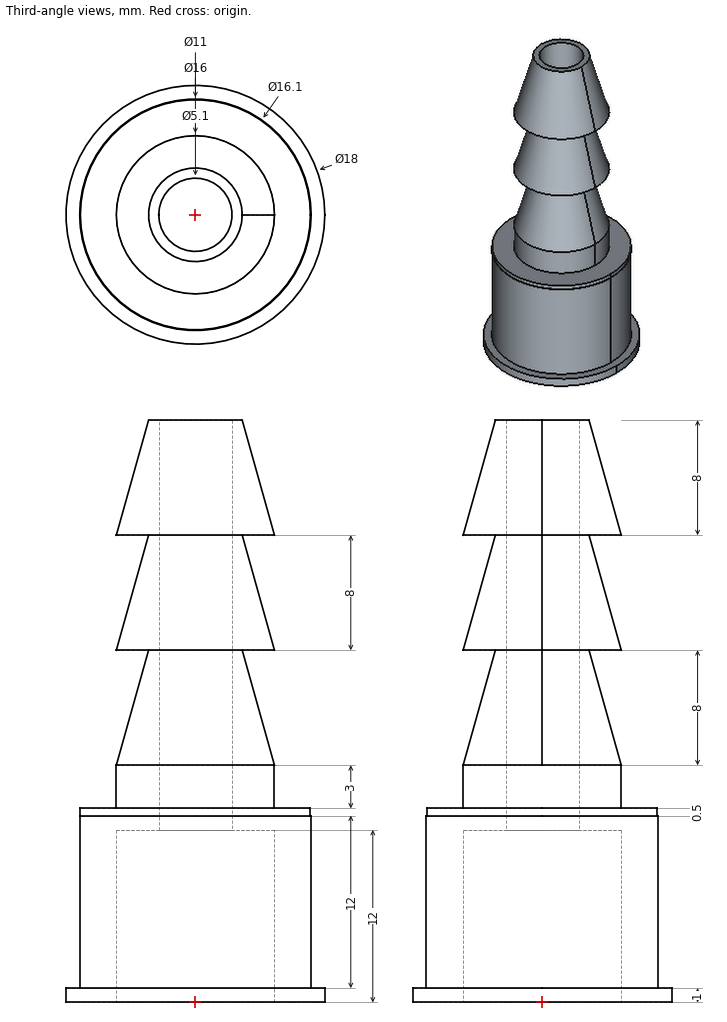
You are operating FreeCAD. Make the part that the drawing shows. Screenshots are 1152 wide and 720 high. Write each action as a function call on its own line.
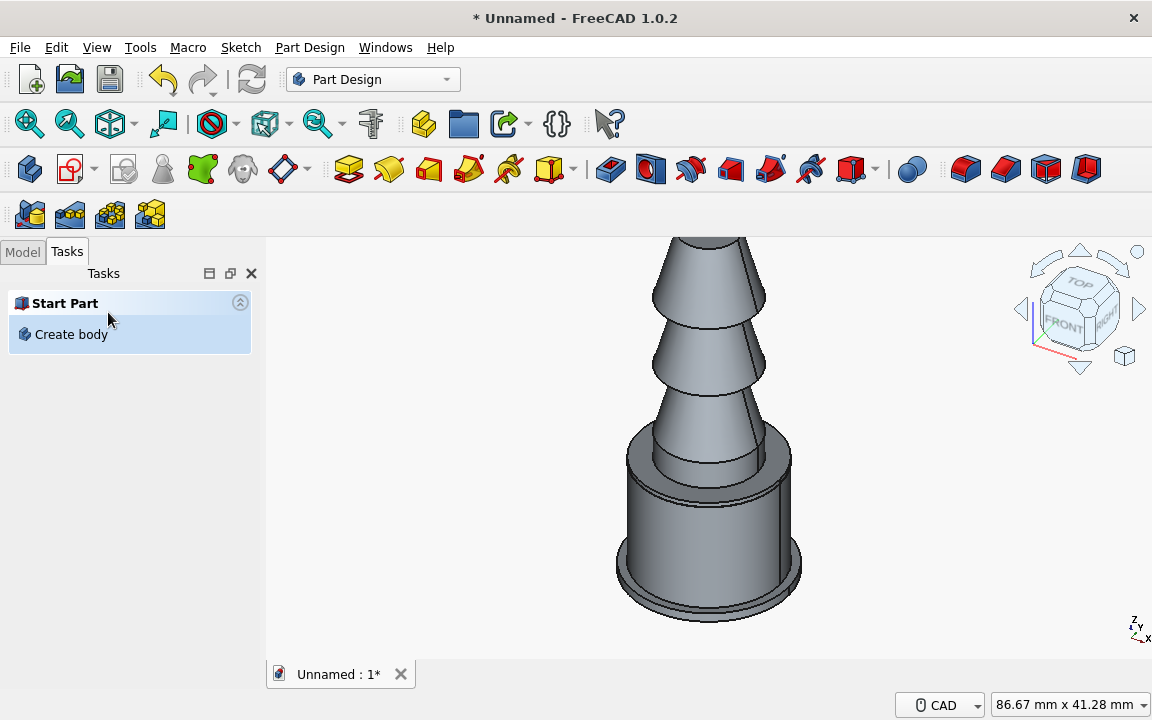
key(v)
key(f)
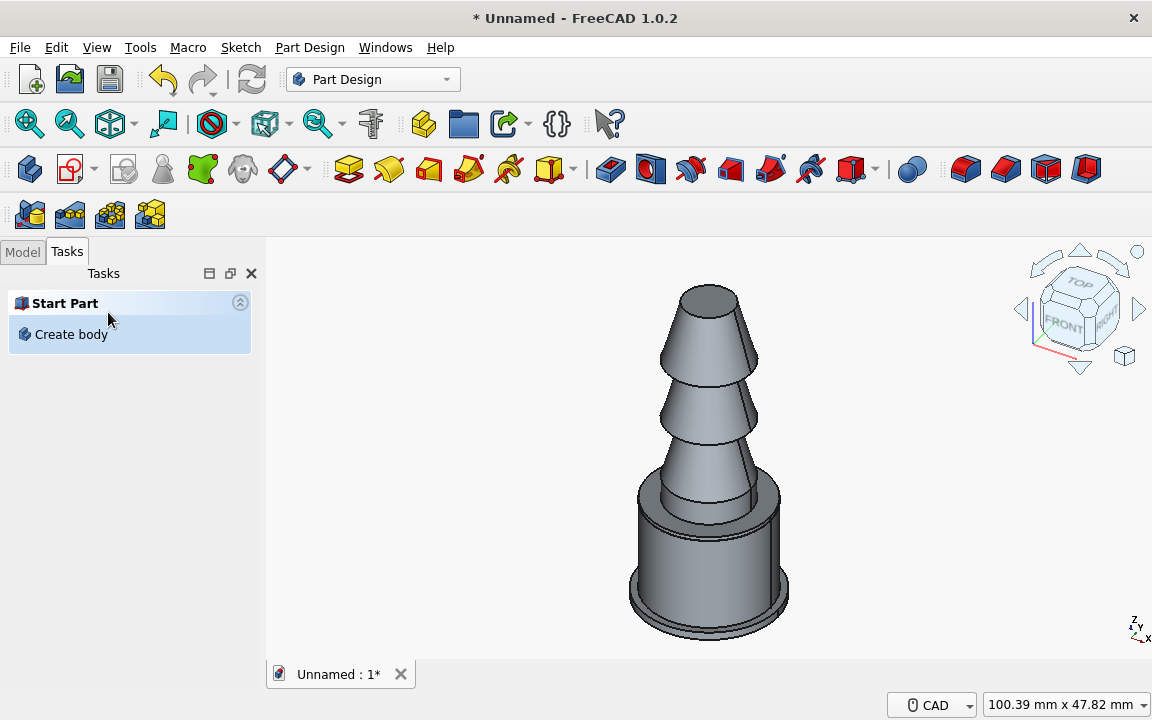
click(70, 170)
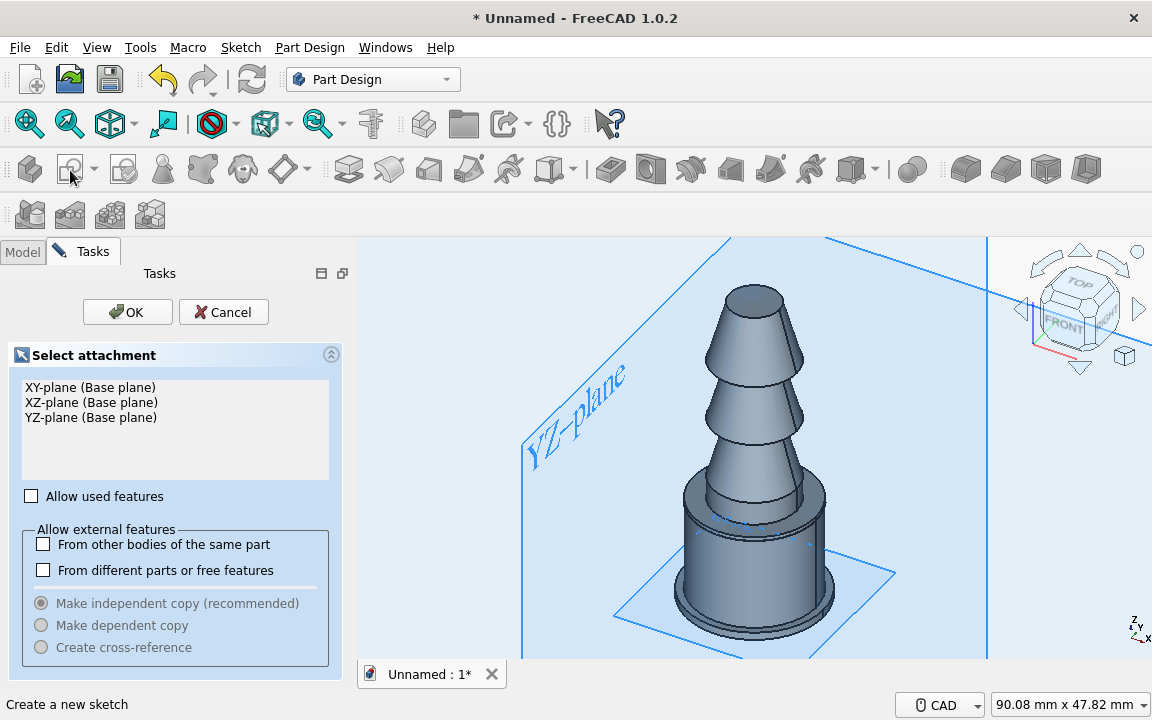
click(82, 388)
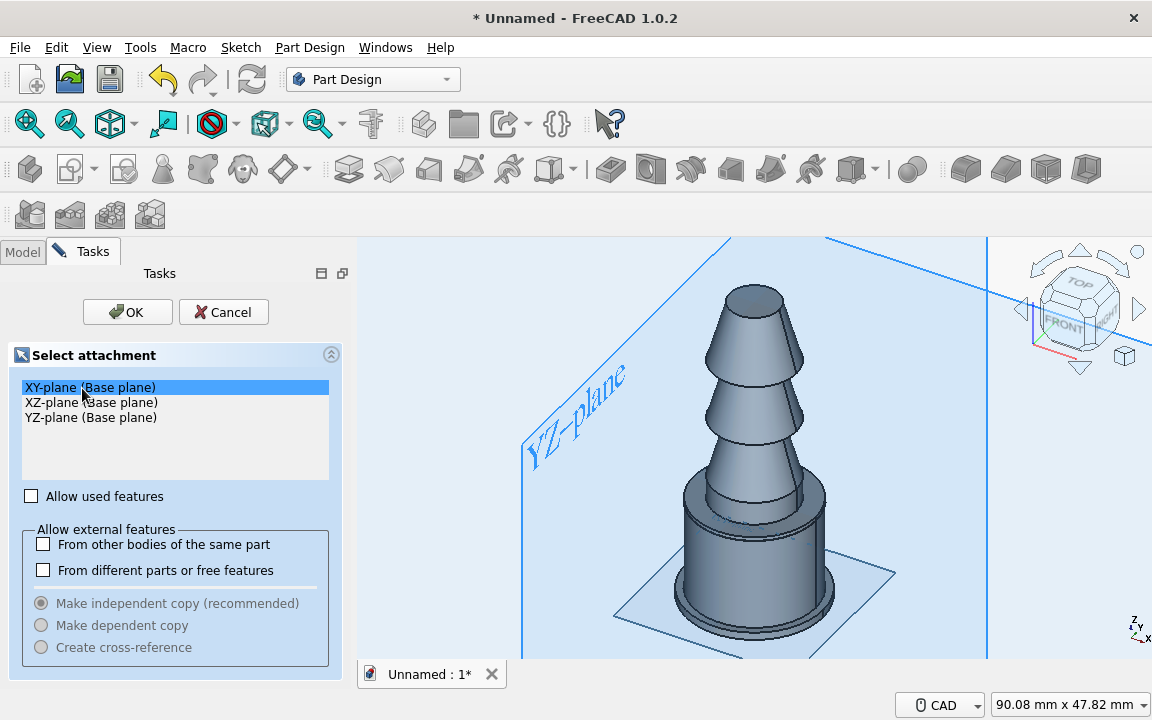
click(128, 312)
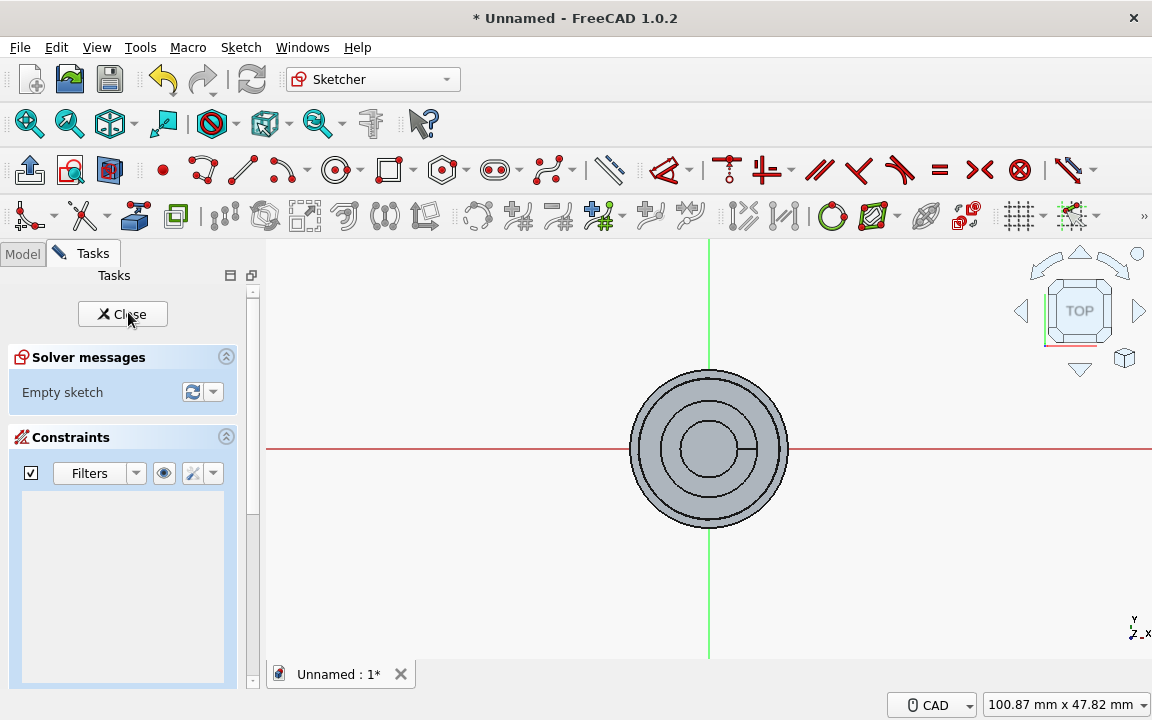
key(q)
key(s)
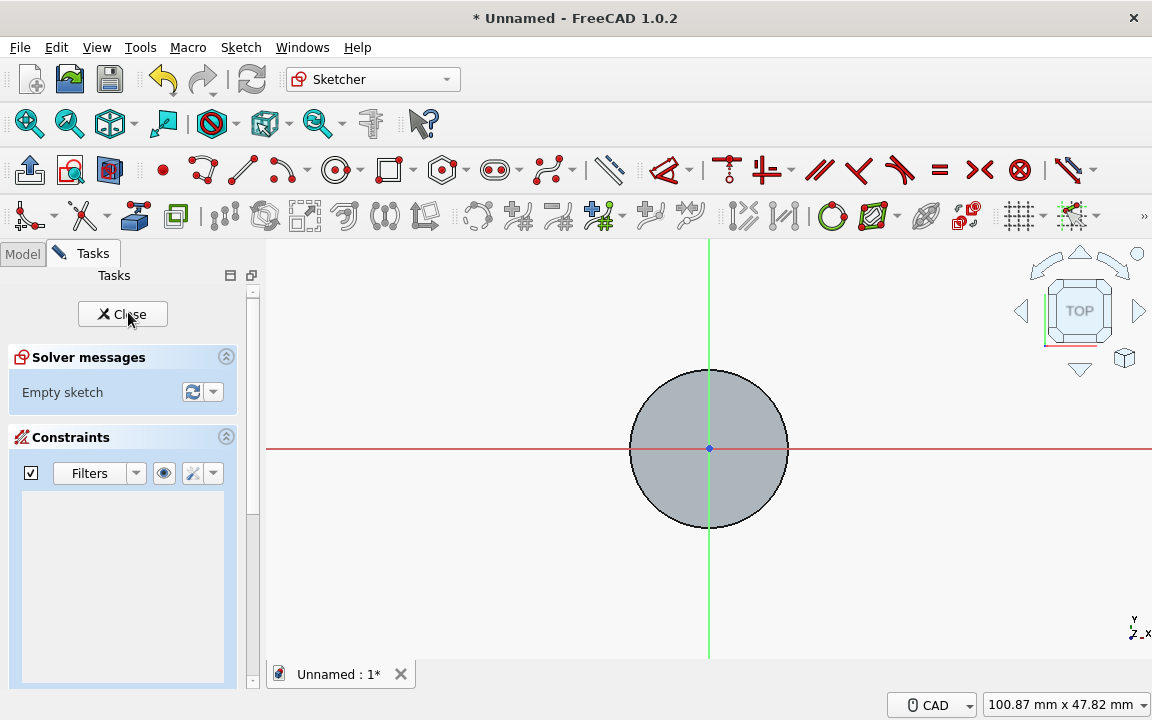
scroll(749, 449, up, 5)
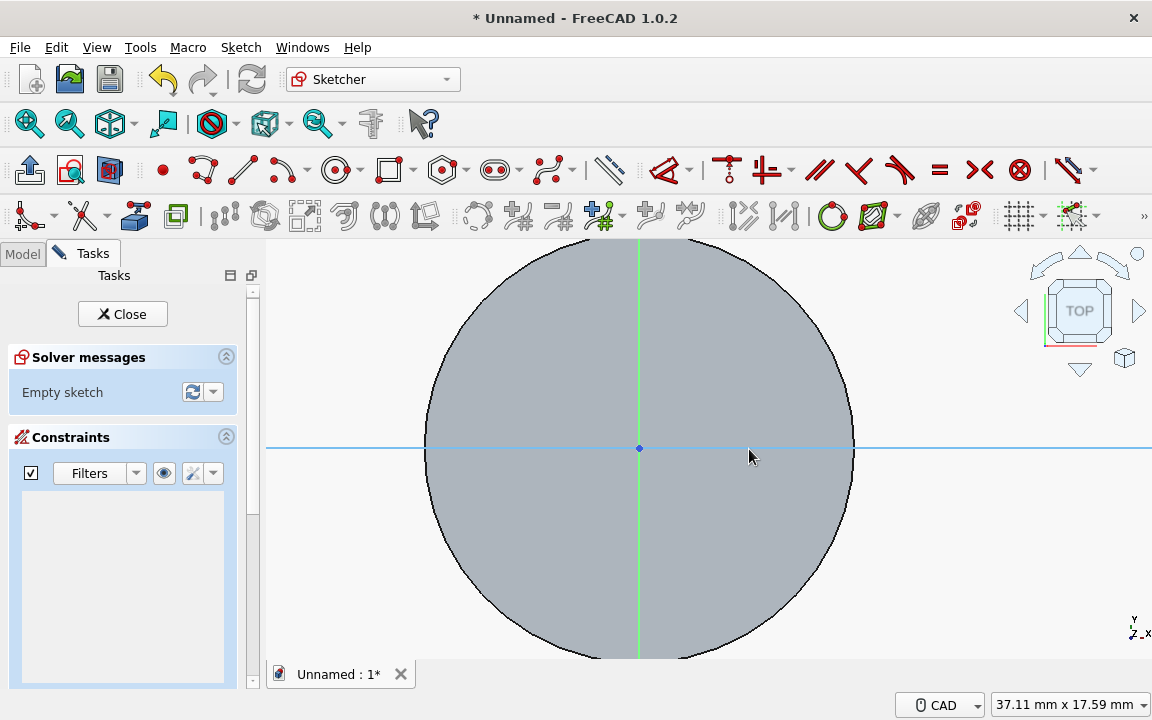
key(g)
key(c)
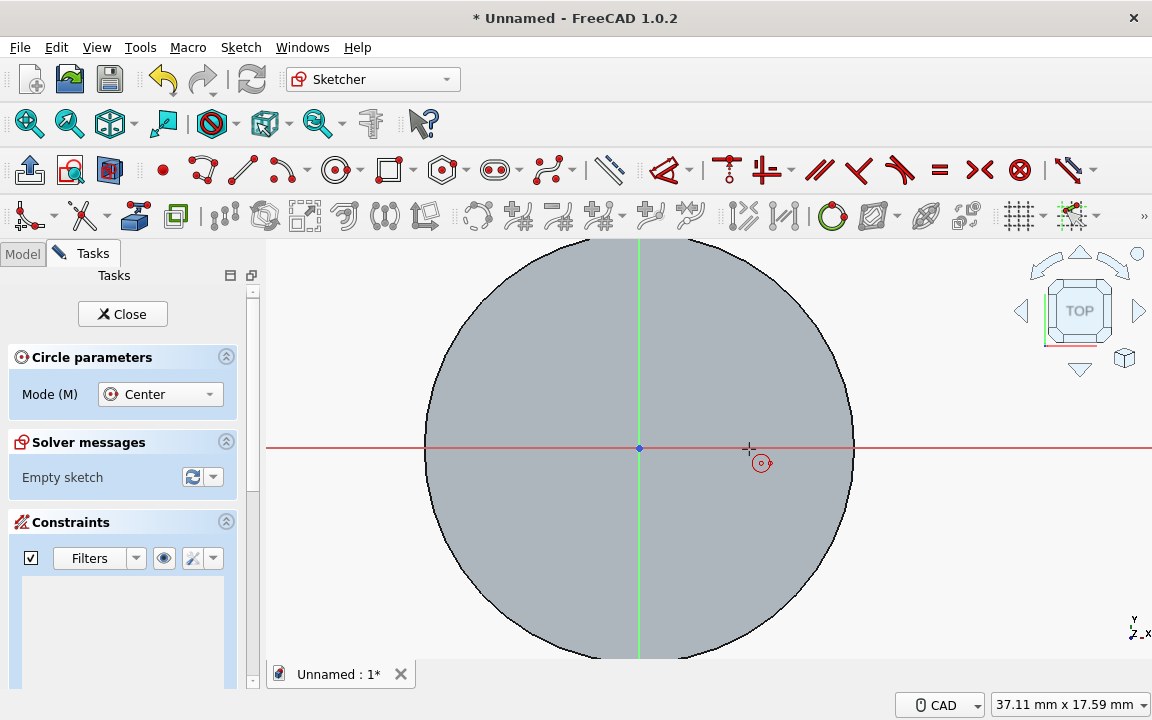
click(639, 448)
click(732, 355)
key(Escape)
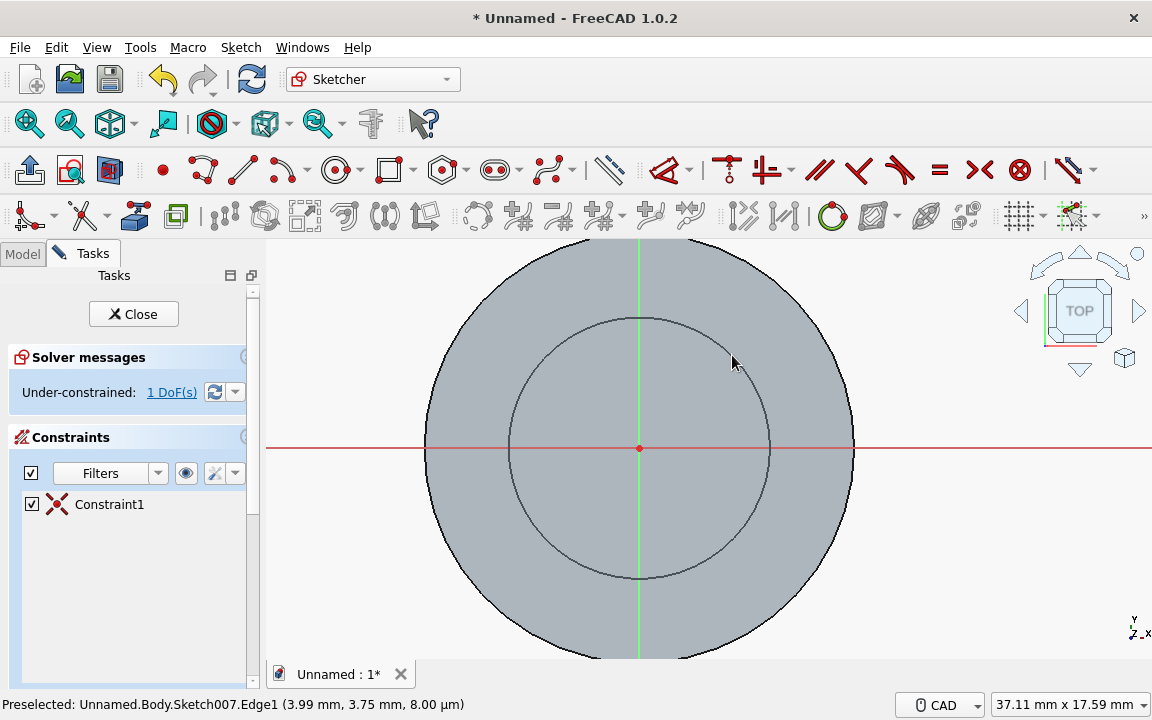
key(d)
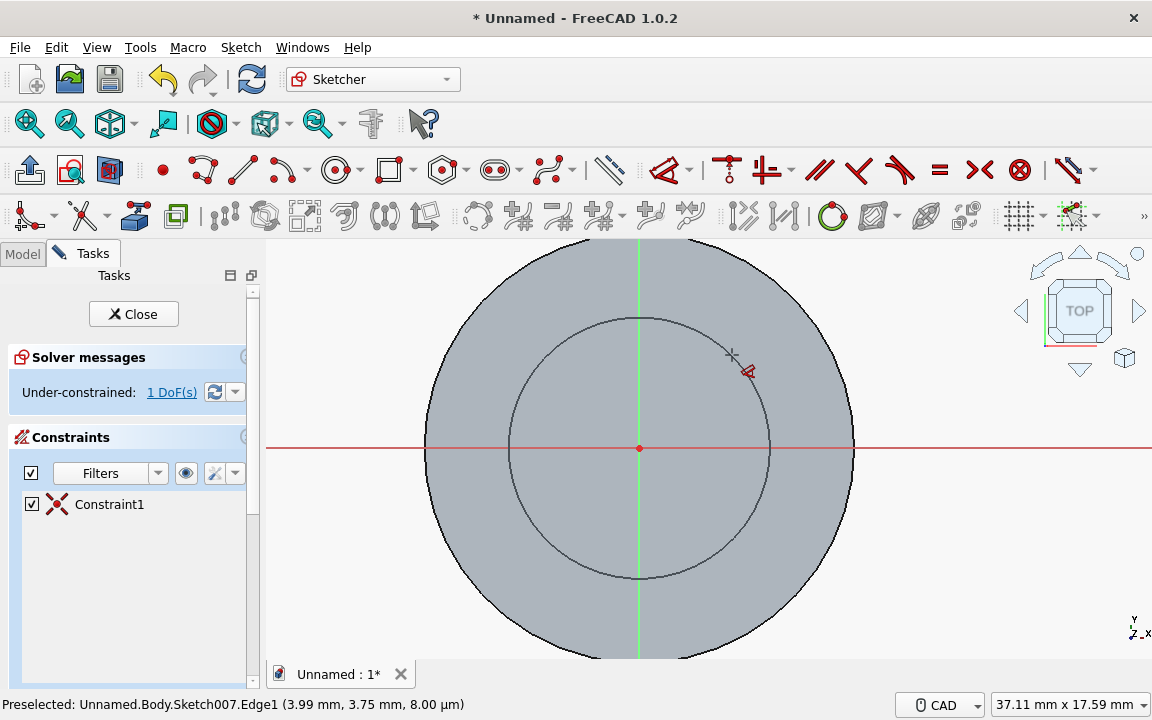
click(731, 355)
click(753, 332)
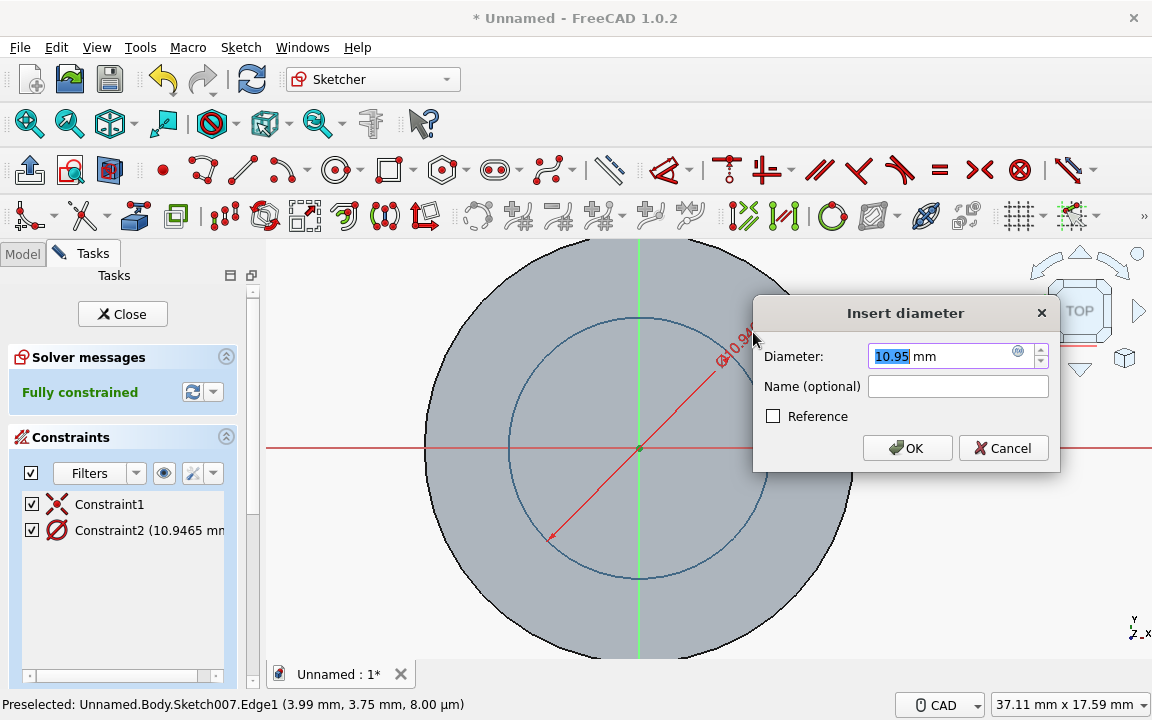
text(11)
key(Return)
key(Escape)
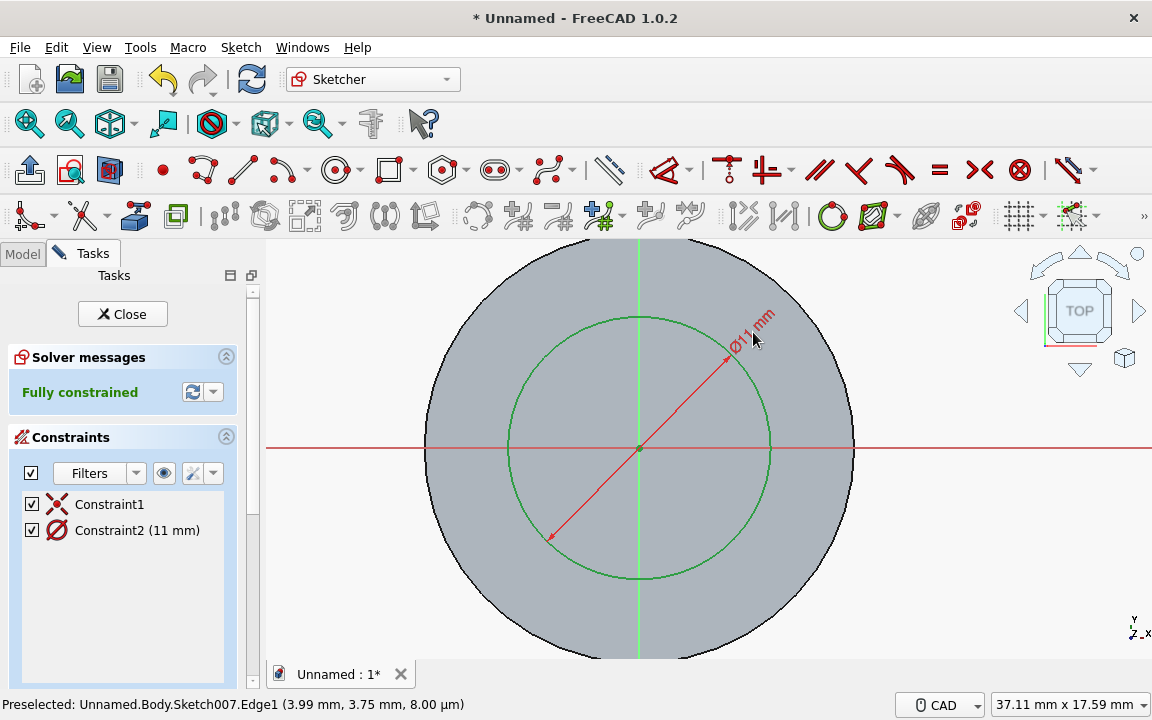
click(123, 314)